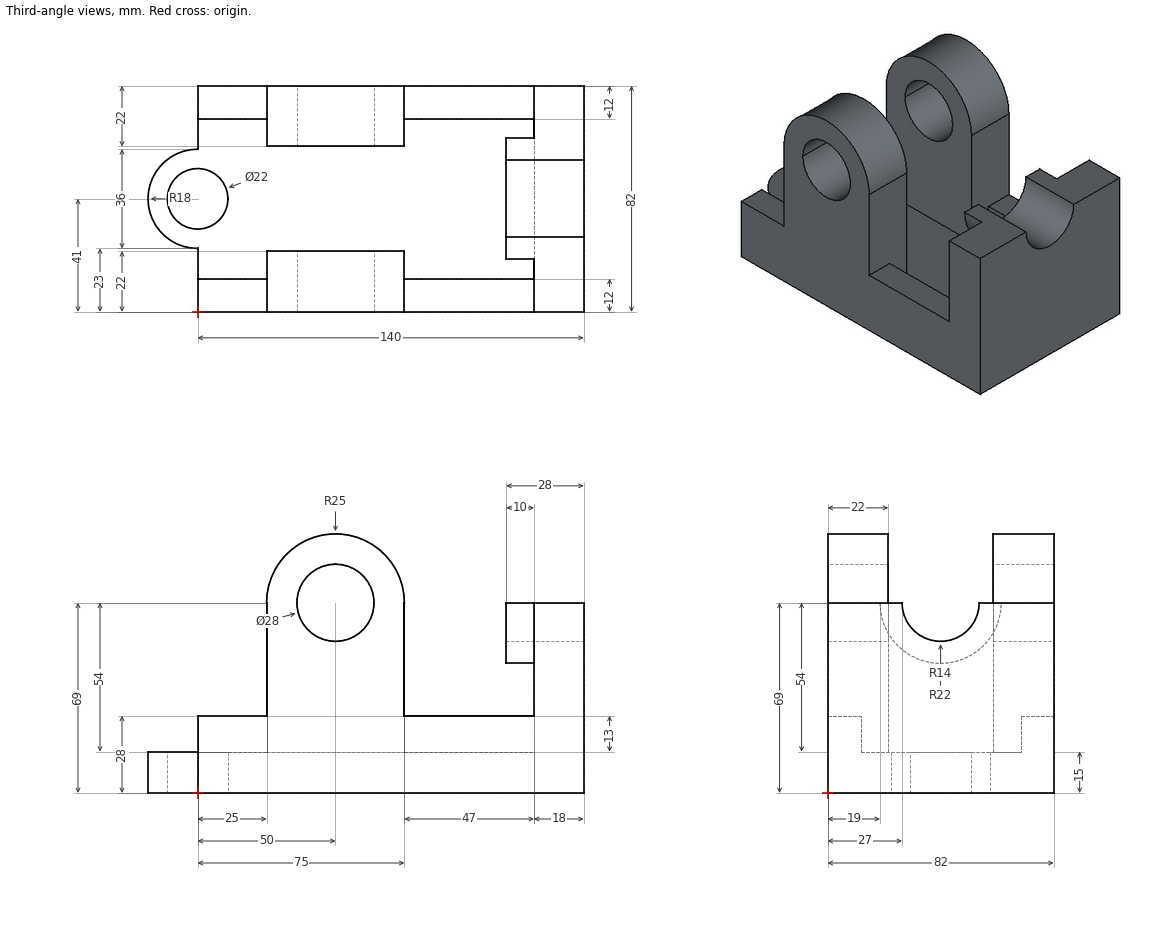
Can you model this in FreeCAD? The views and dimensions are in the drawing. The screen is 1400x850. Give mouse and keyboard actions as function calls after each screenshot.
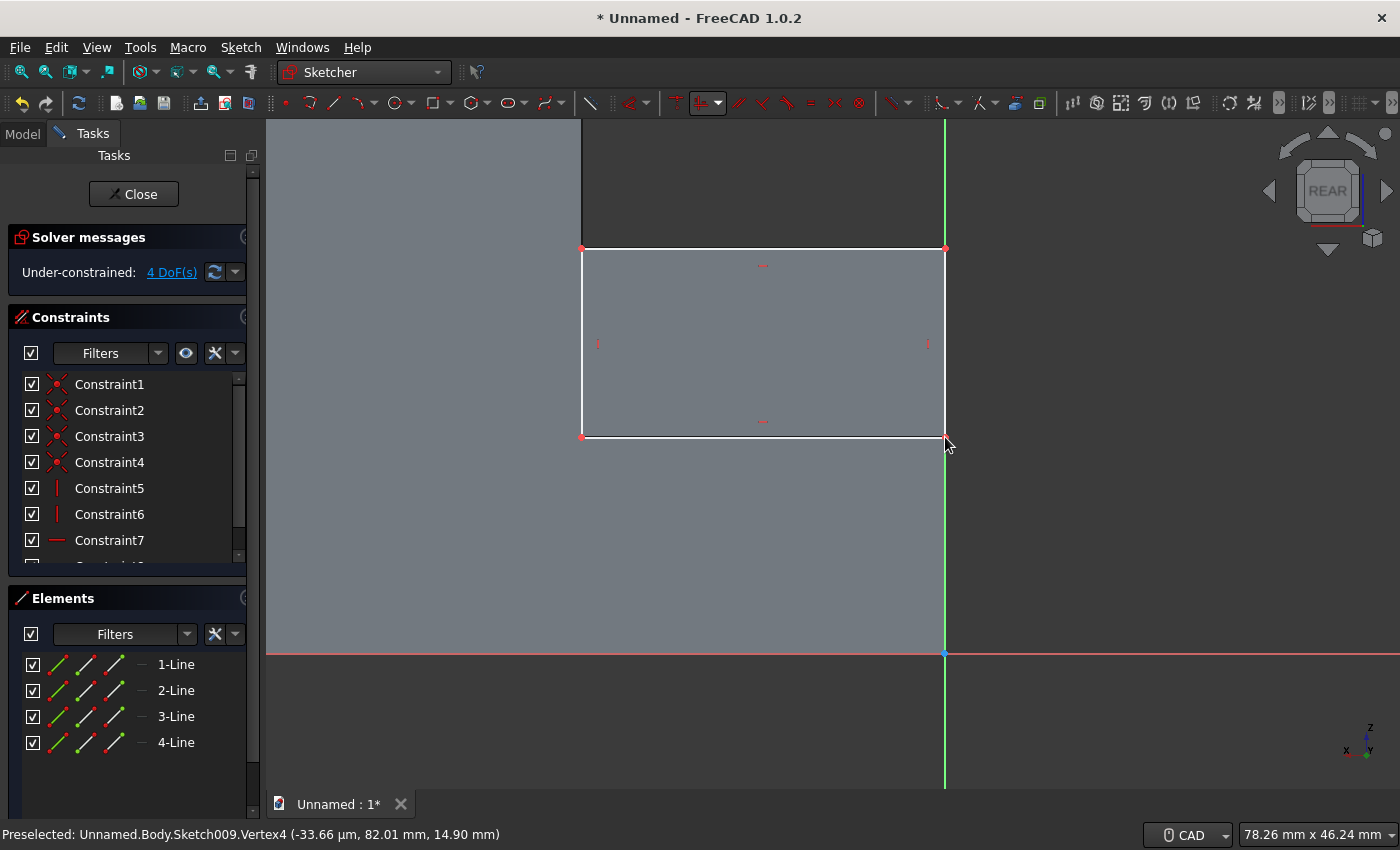
click(945, 438)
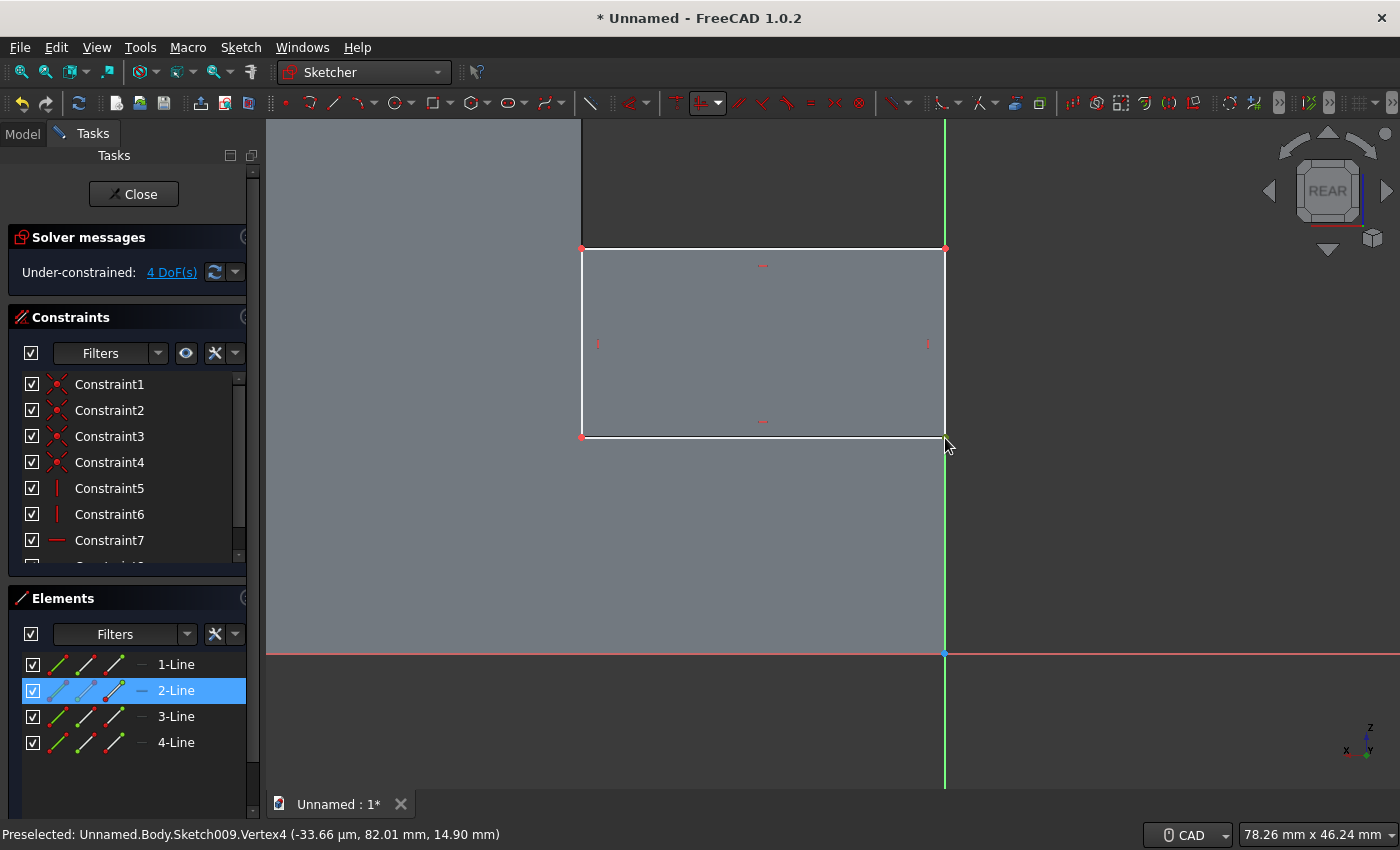
click(945, 717)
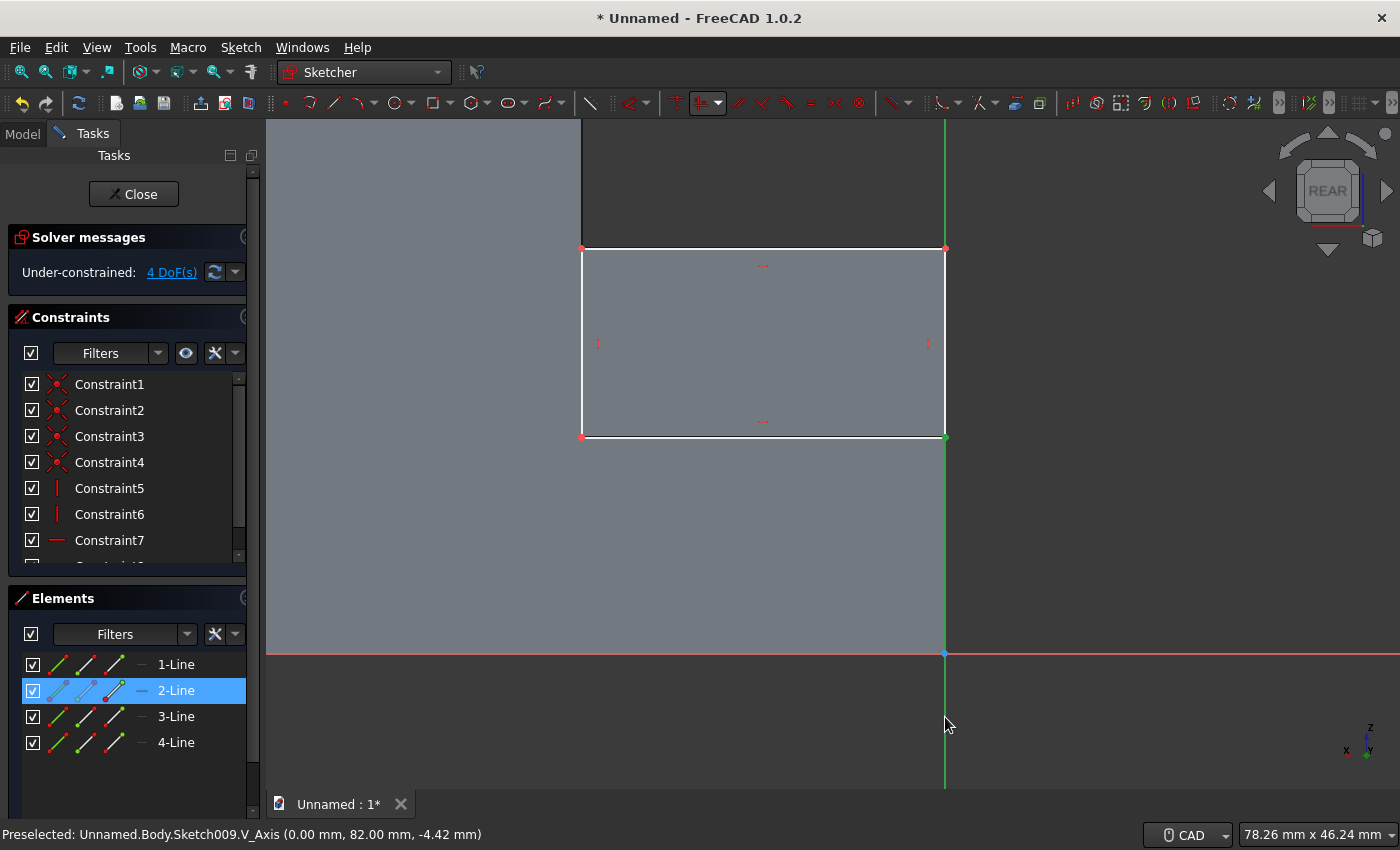
click(676, 104)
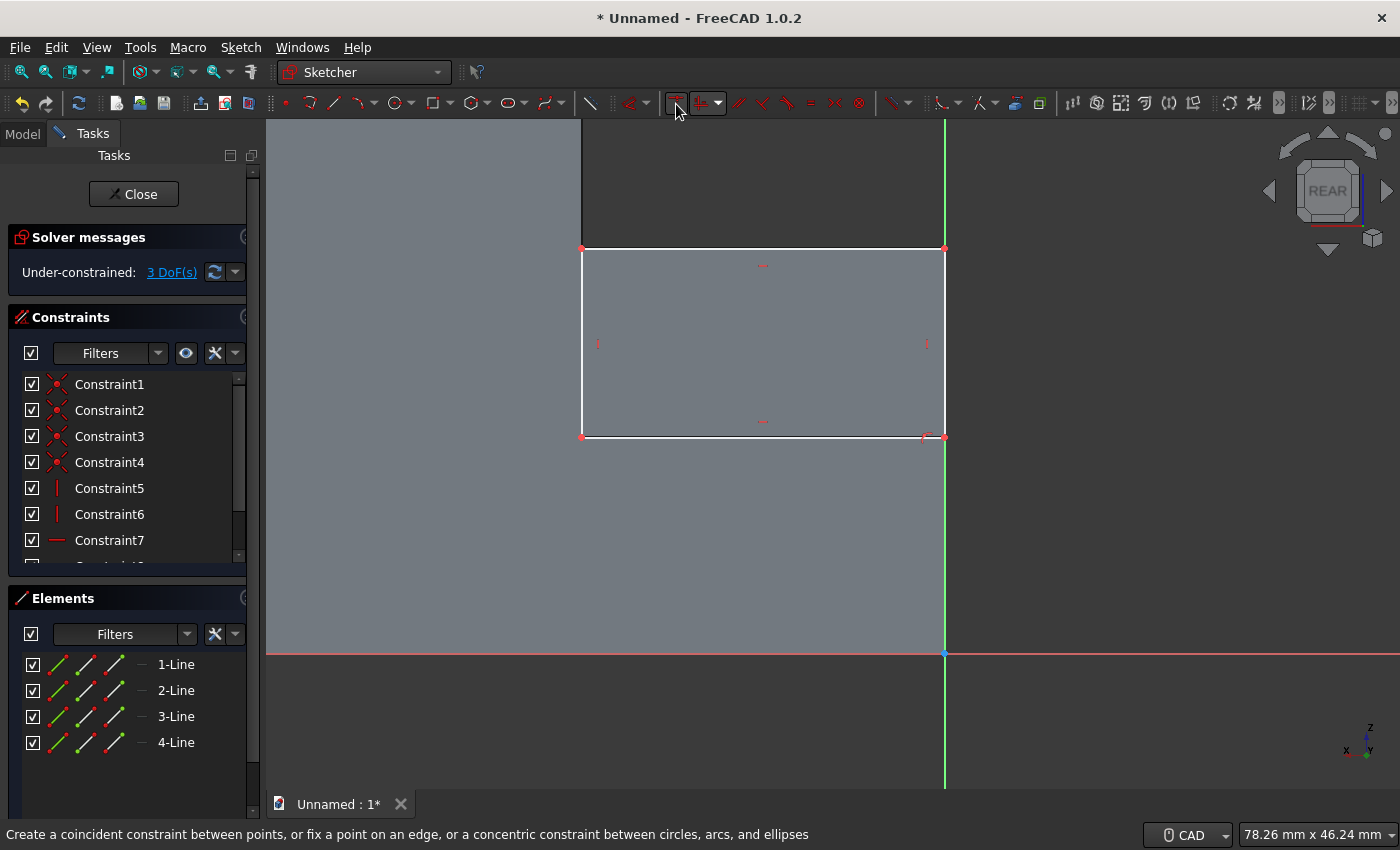
click(630, 104)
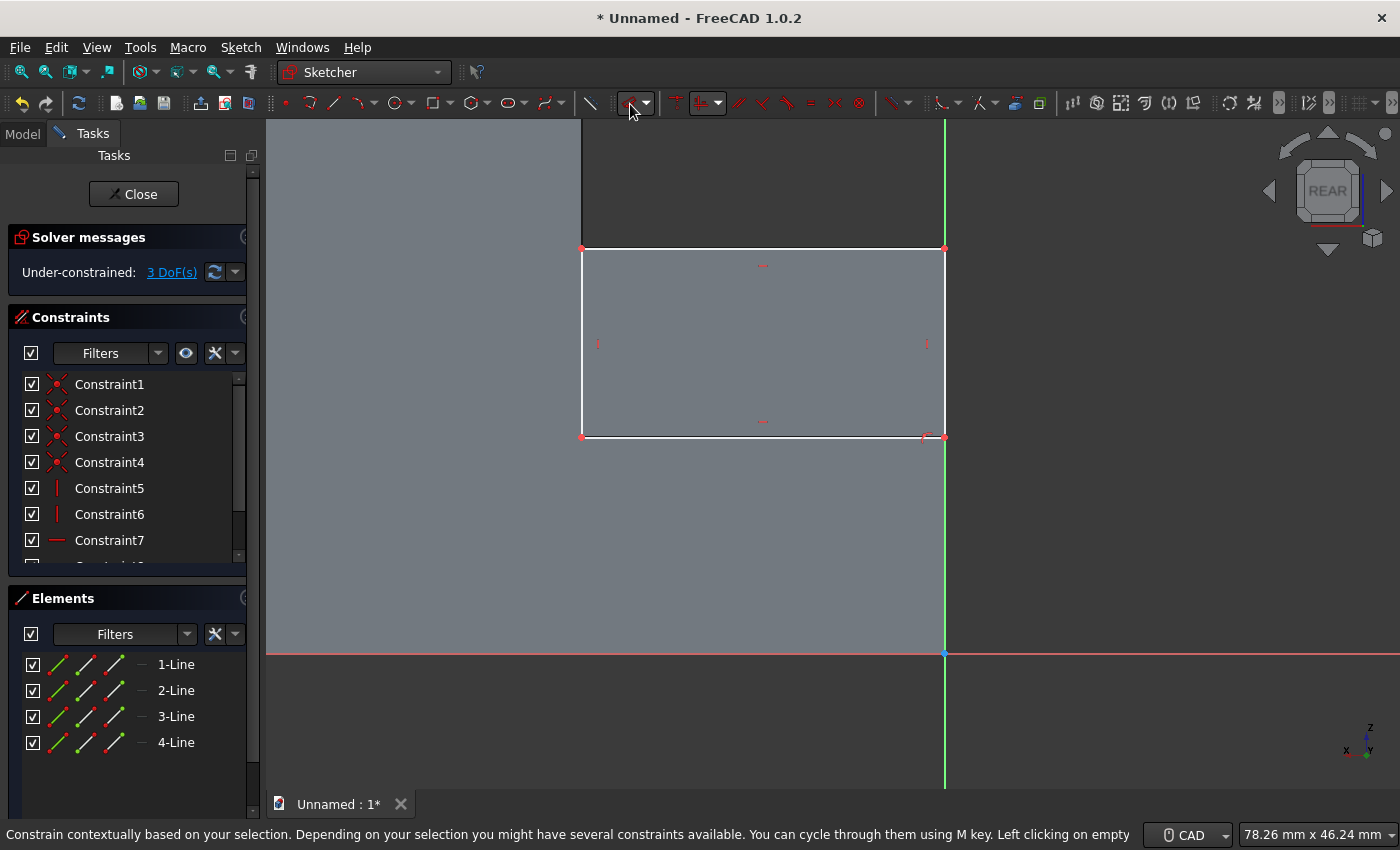
click(582, 306)
click(548, 344)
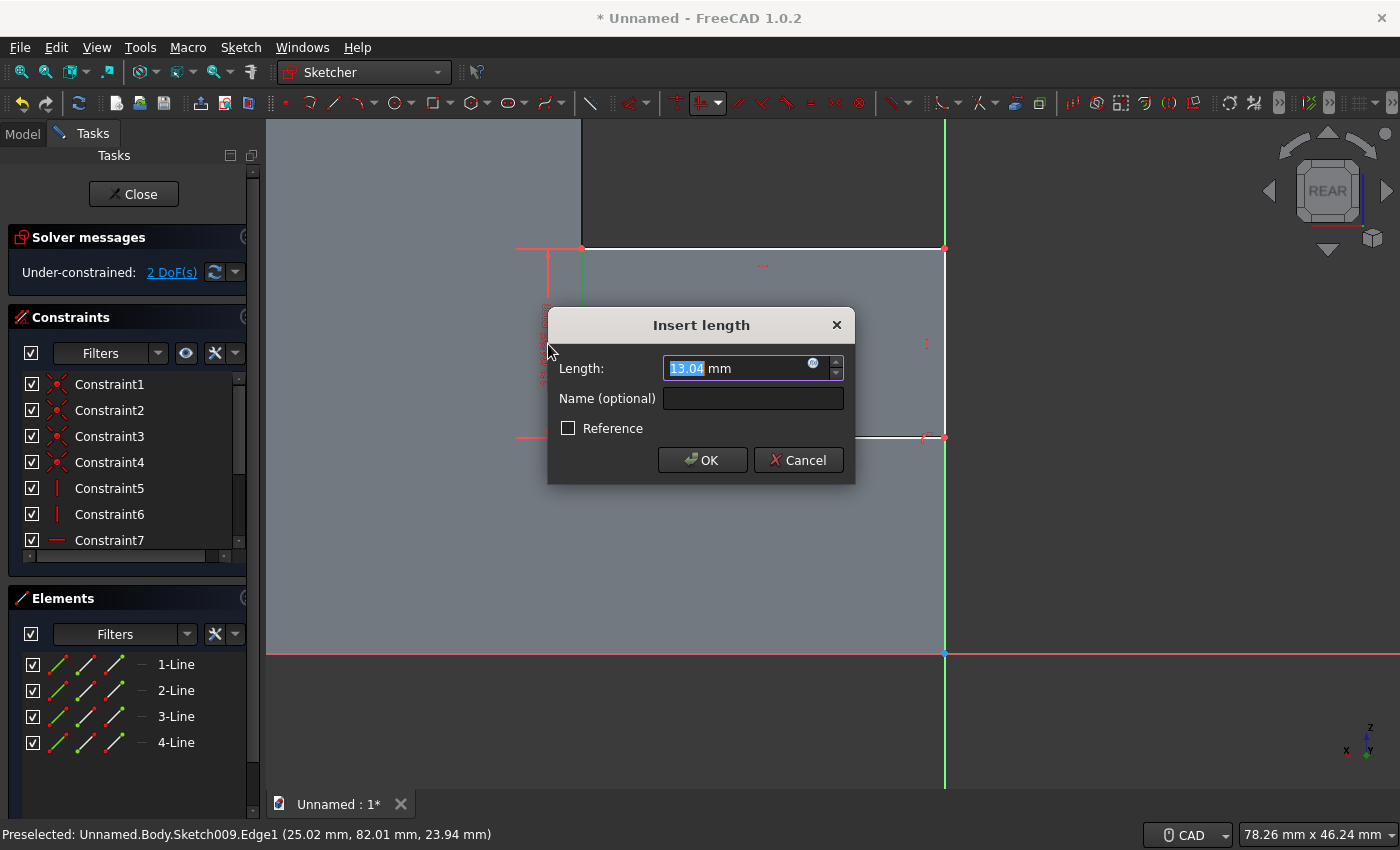
text(13)
key(Return)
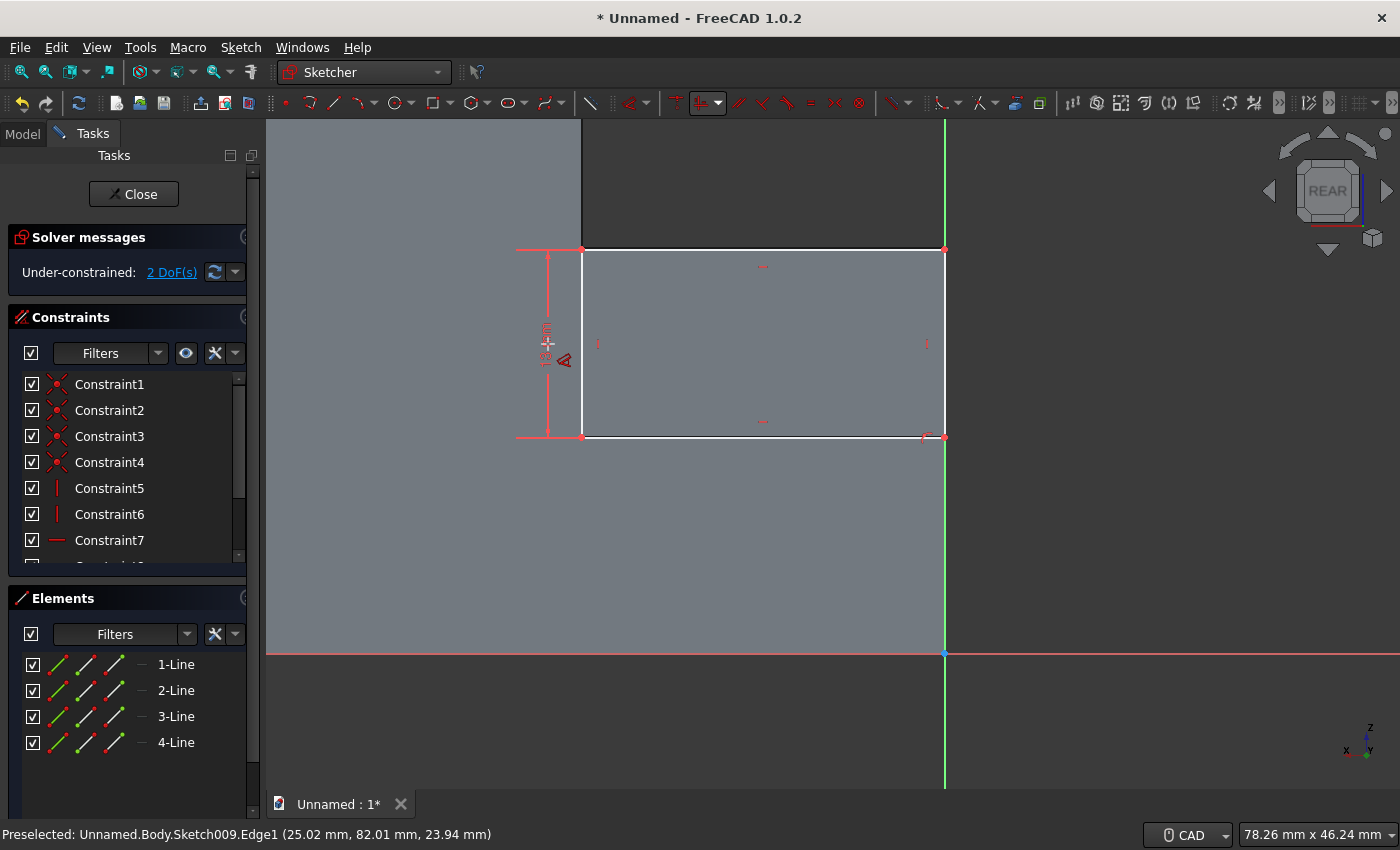
click(691, 438)
click(763, 404)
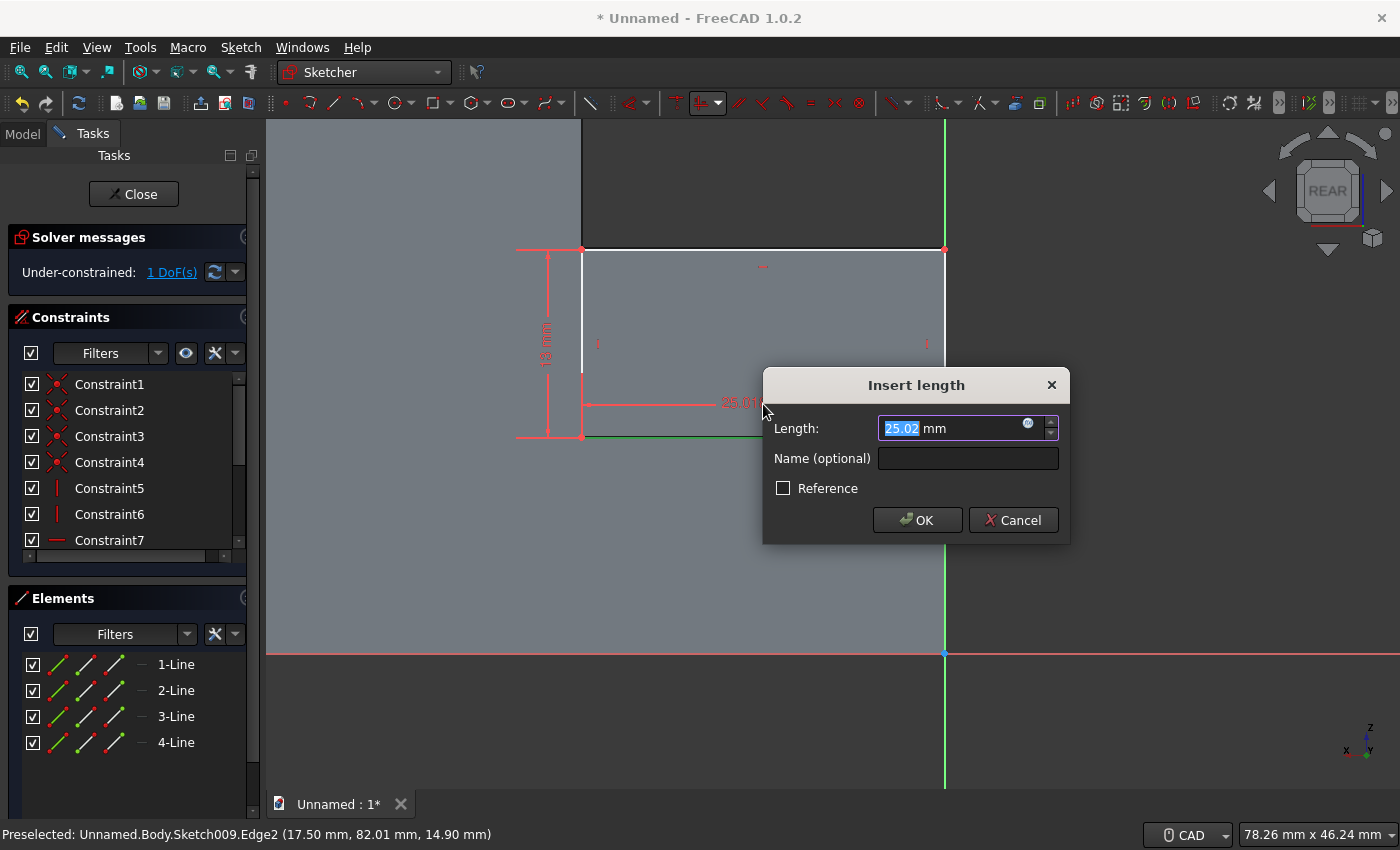
text(25)
key(Return)